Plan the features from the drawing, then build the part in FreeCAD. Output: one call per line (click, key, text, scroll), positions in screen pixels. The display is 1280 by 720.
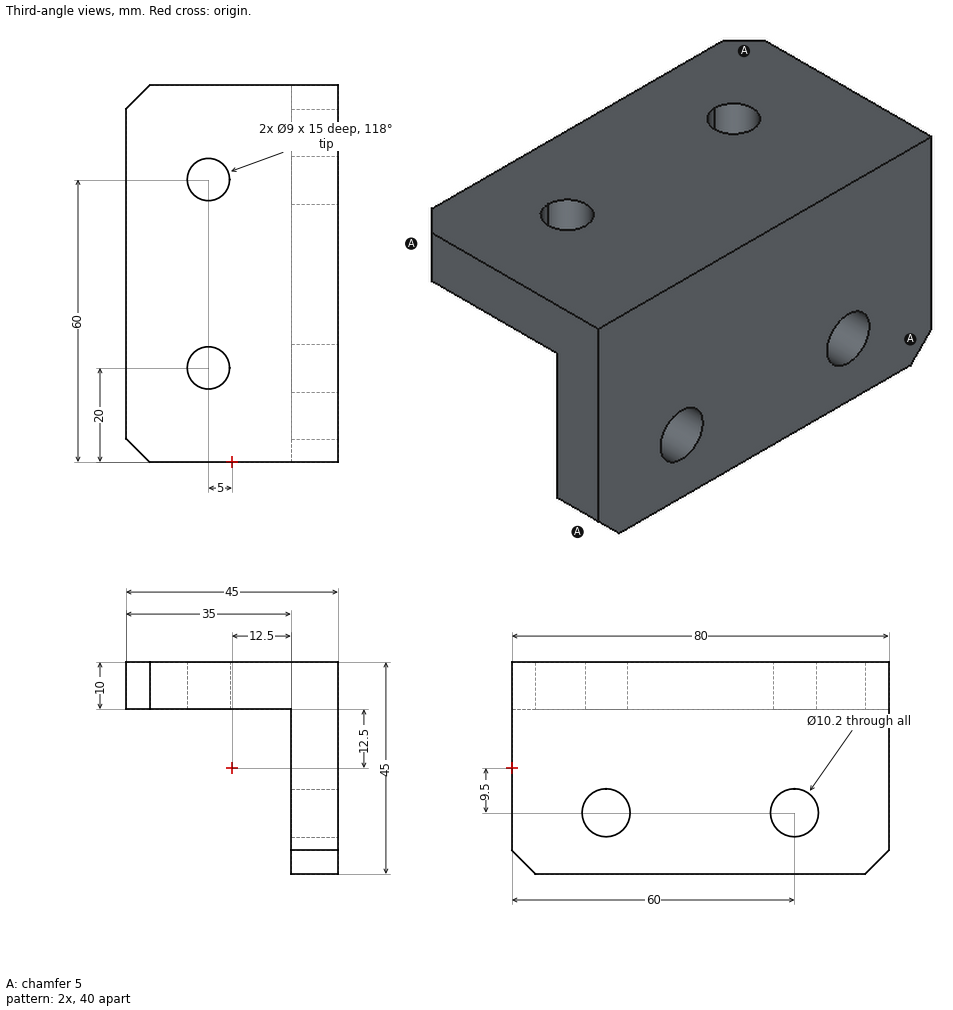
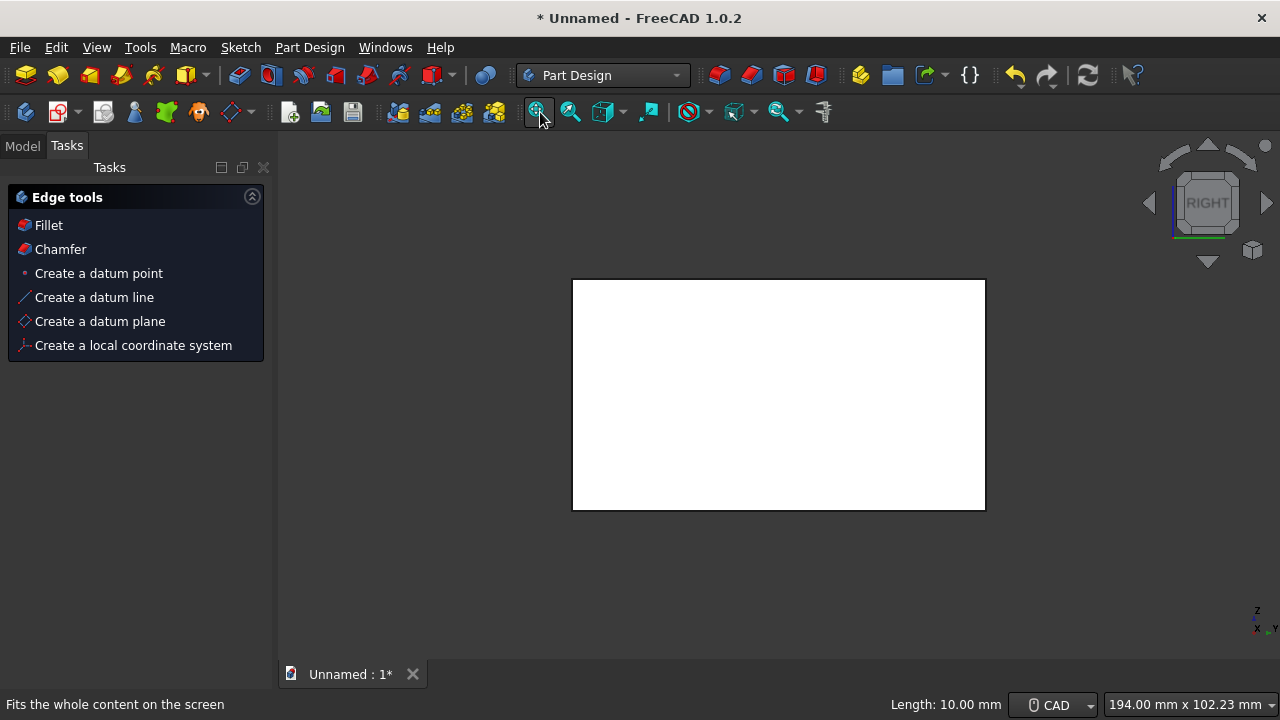
key(5)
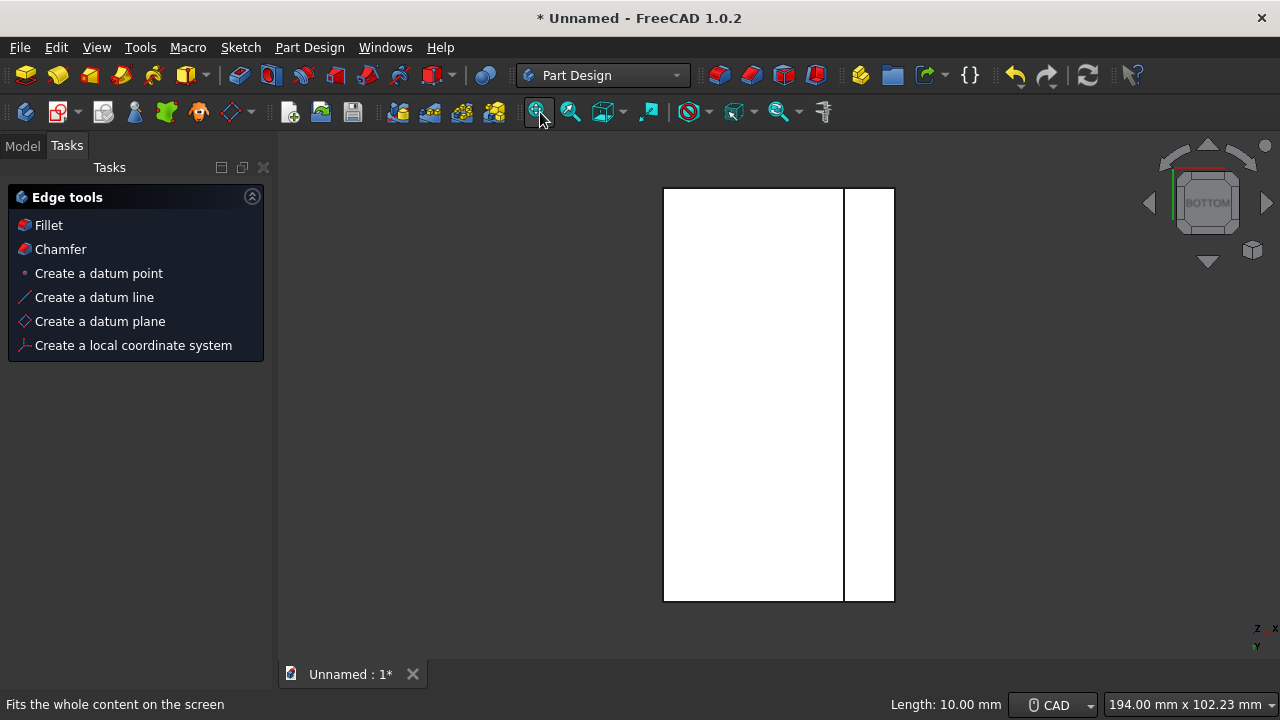
click(869, 187, ctrl)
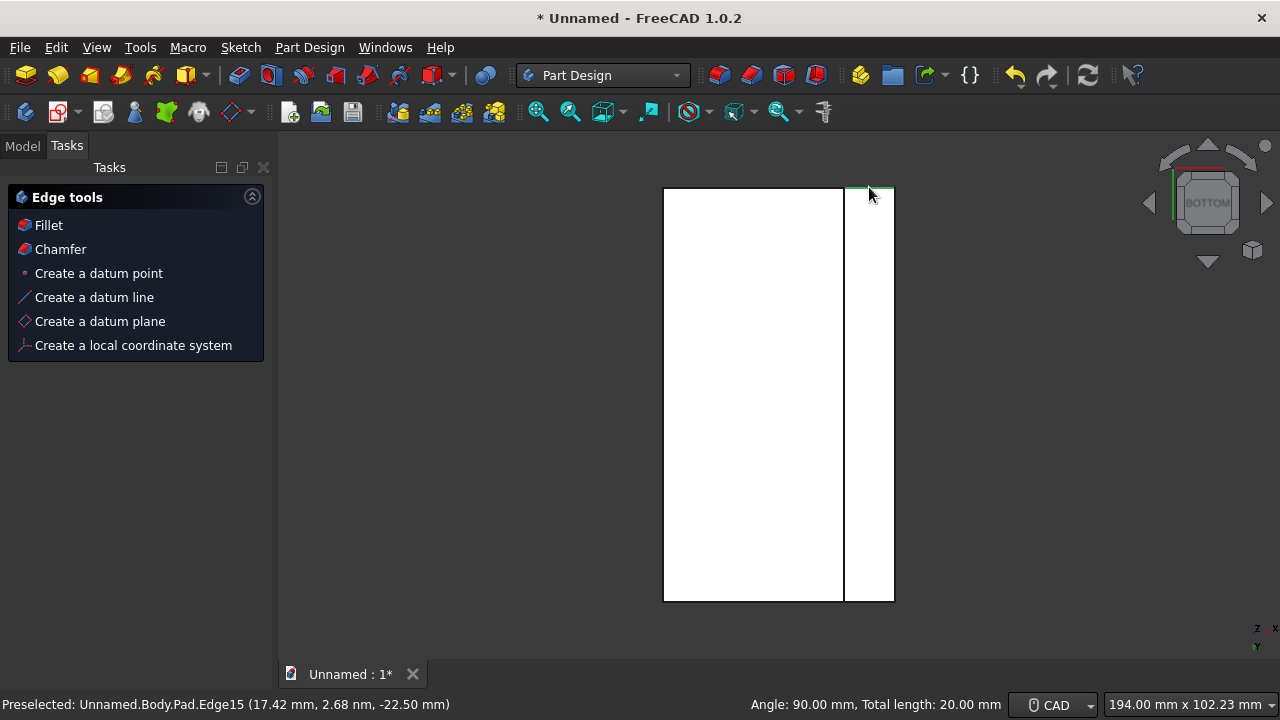
key(4)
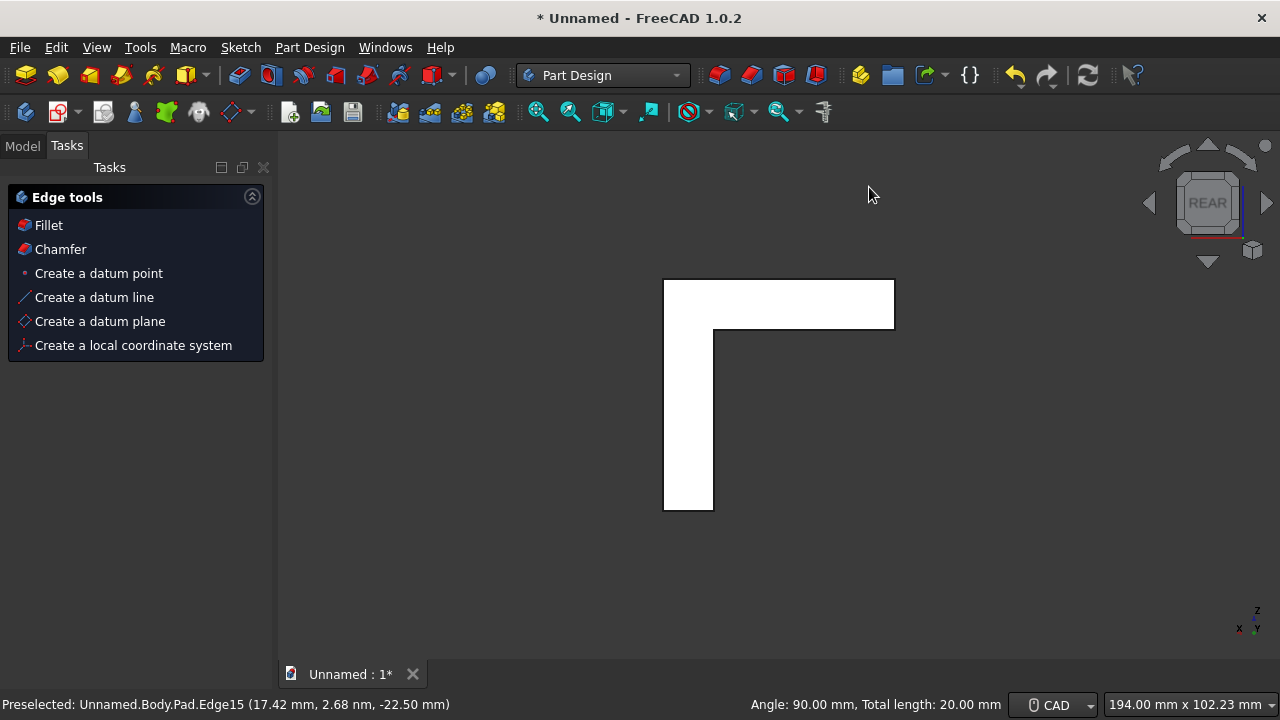
click(540, 112)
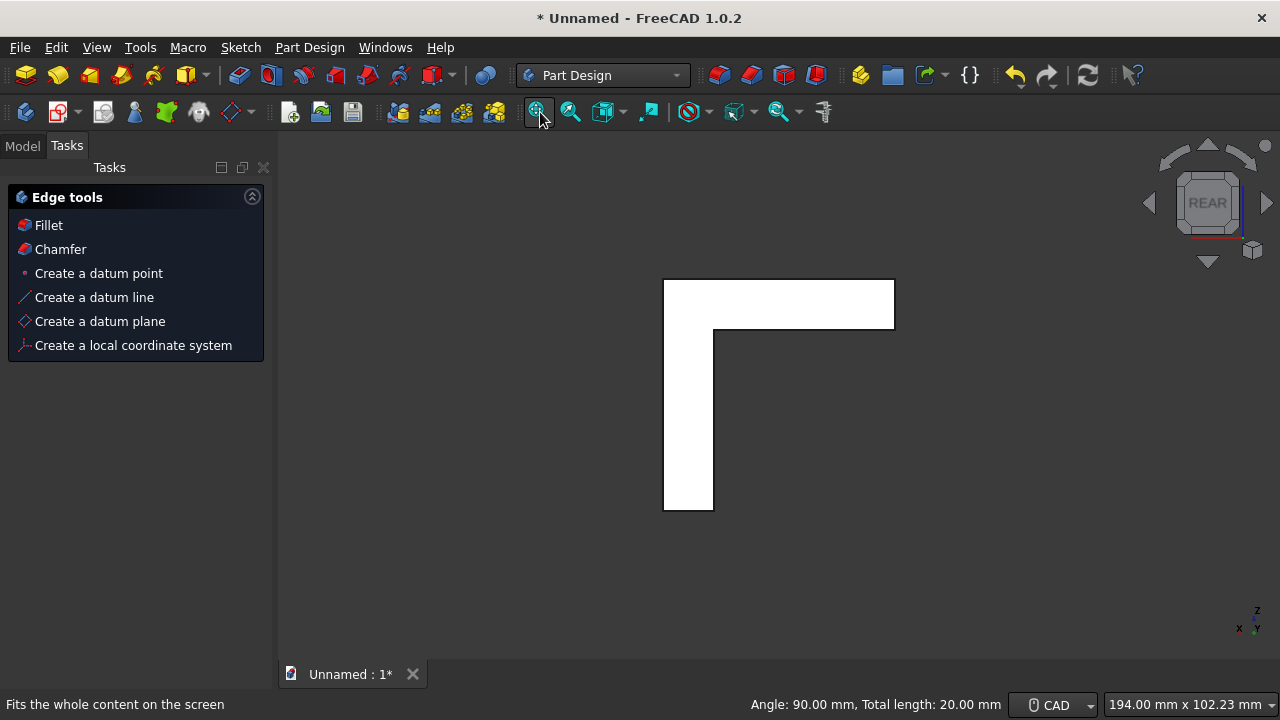
click(895, 304, ctrl)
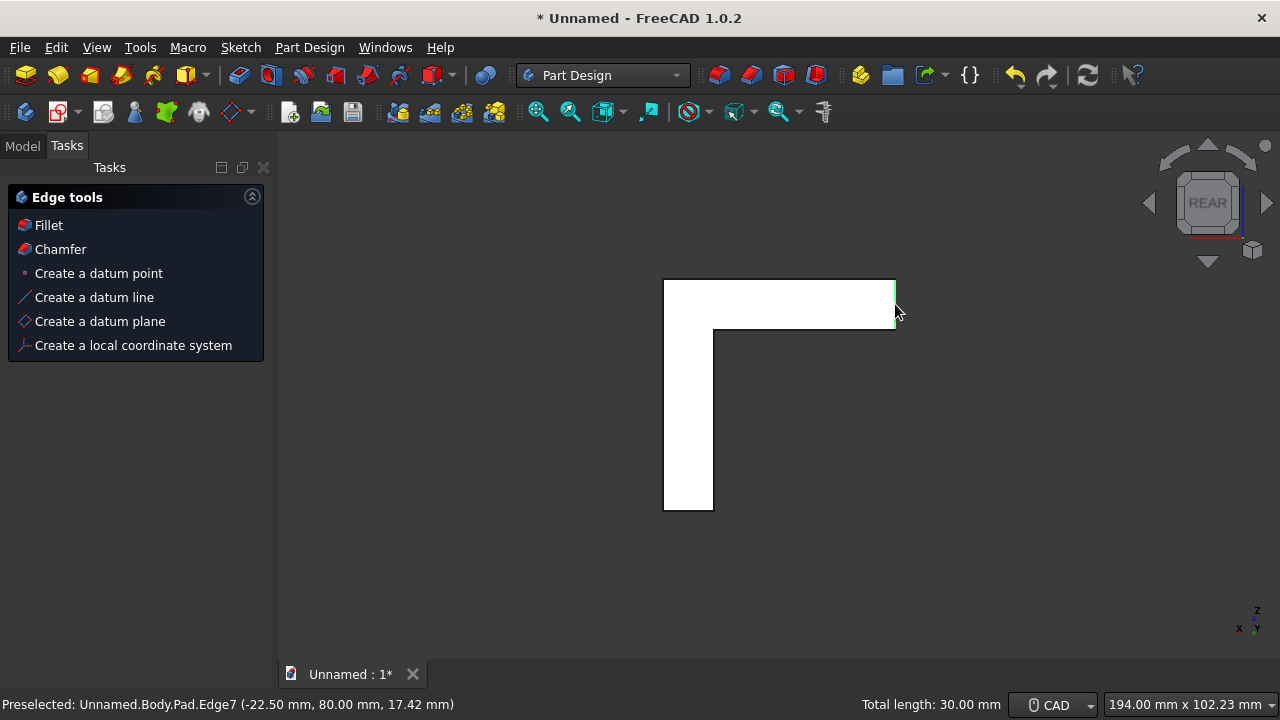
click(689, 510, ctrl)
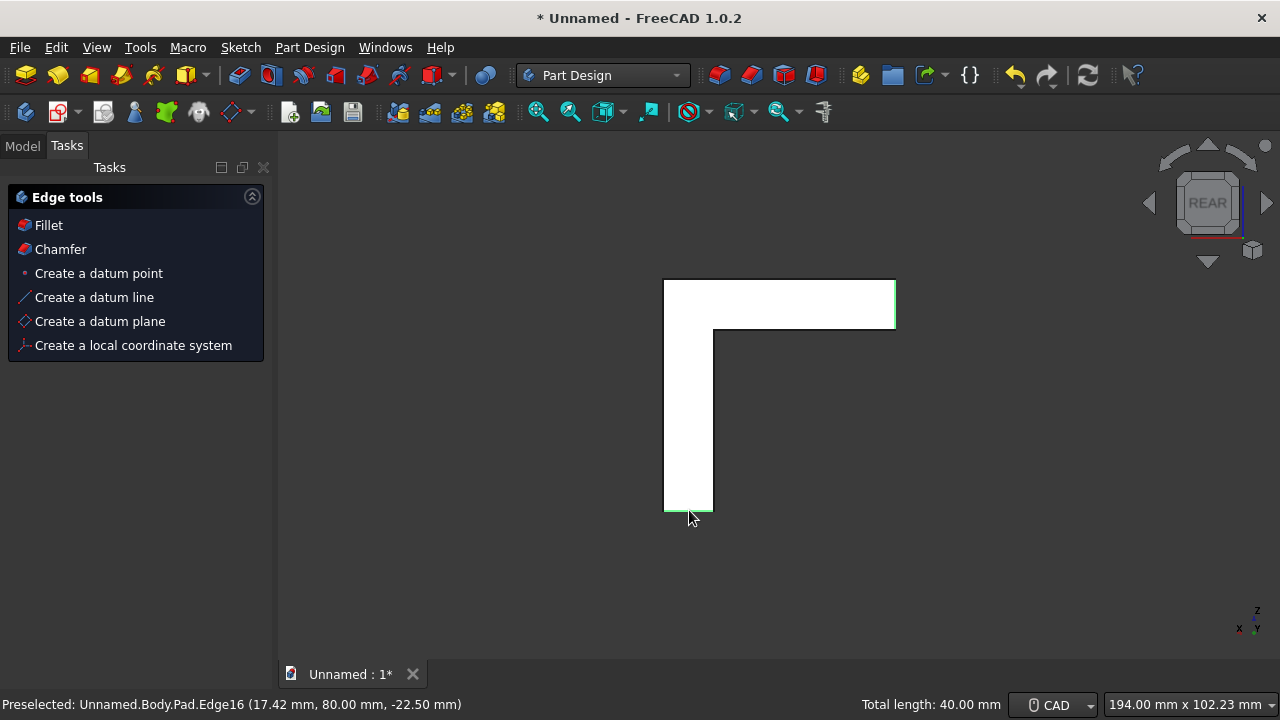
click(752, 76)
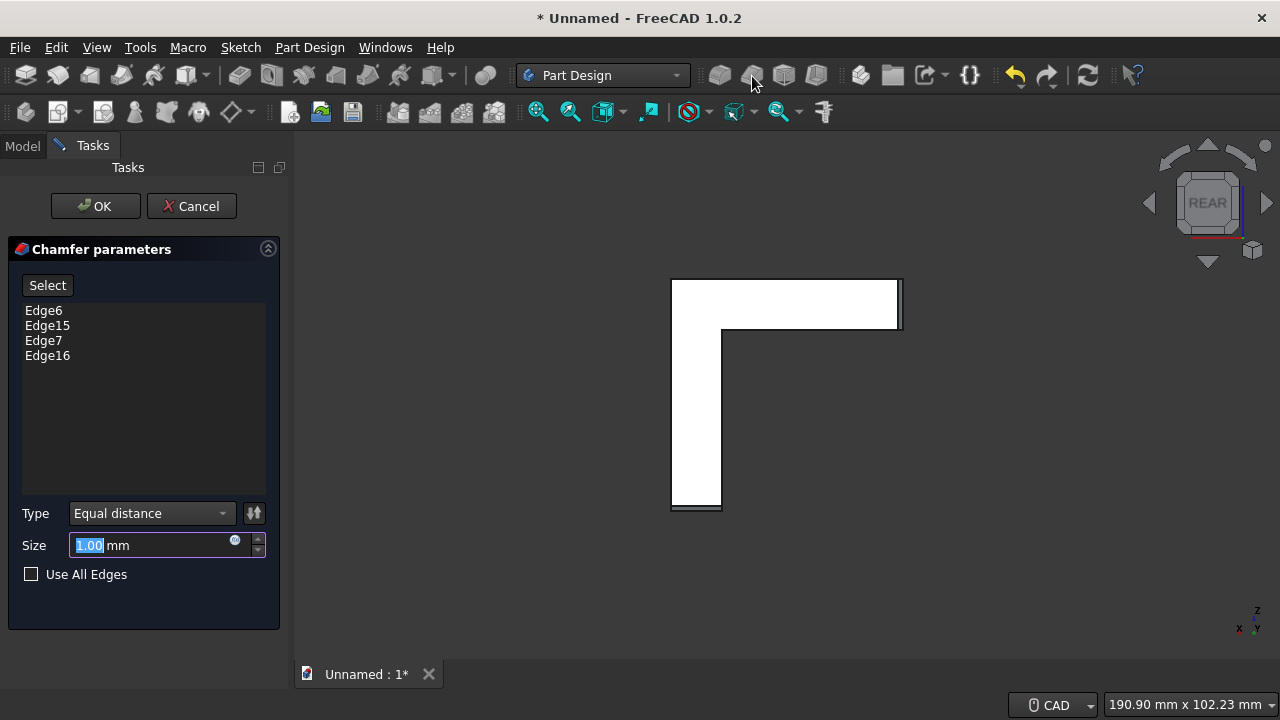
text(5)
key(Tab)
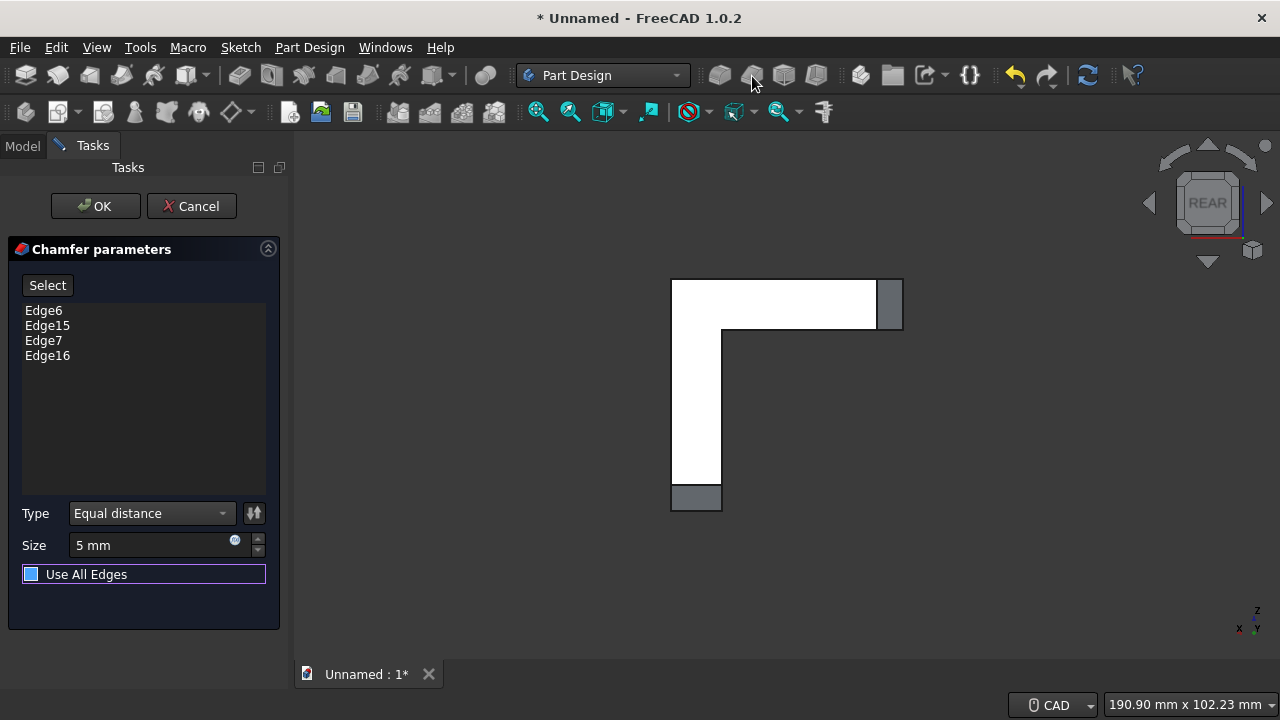
click(96, 206)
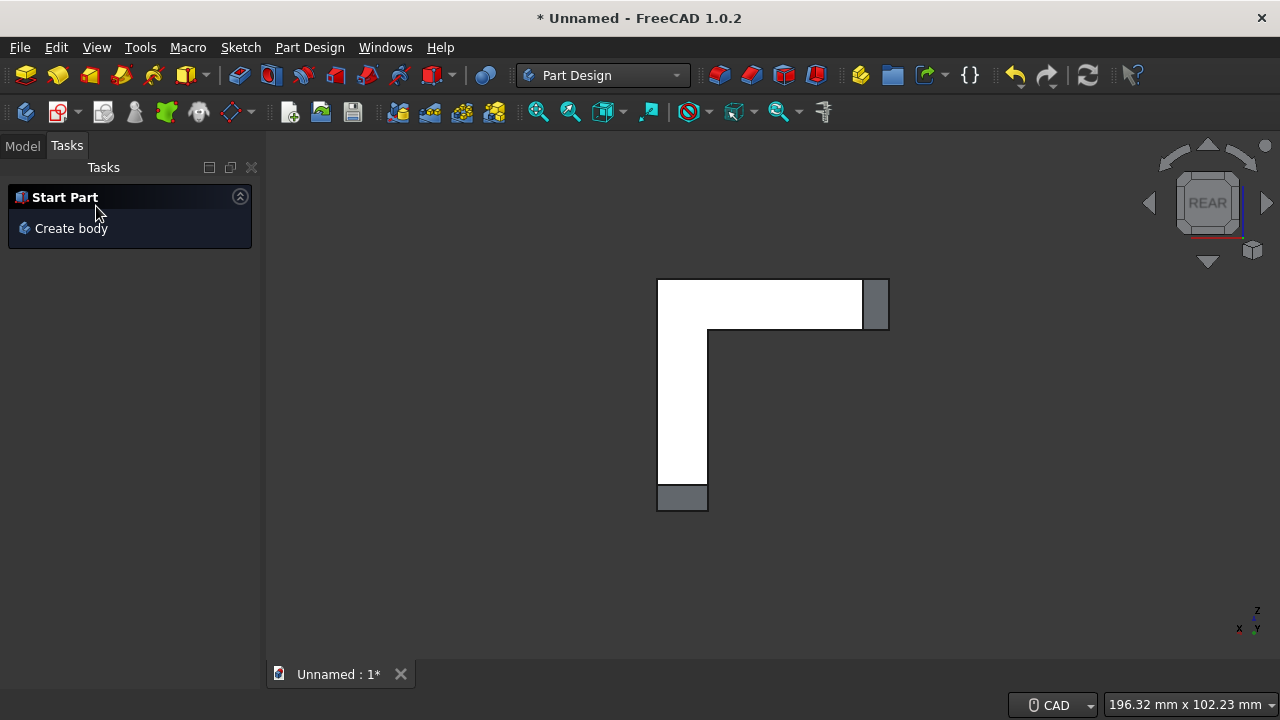
key(v)
key(f)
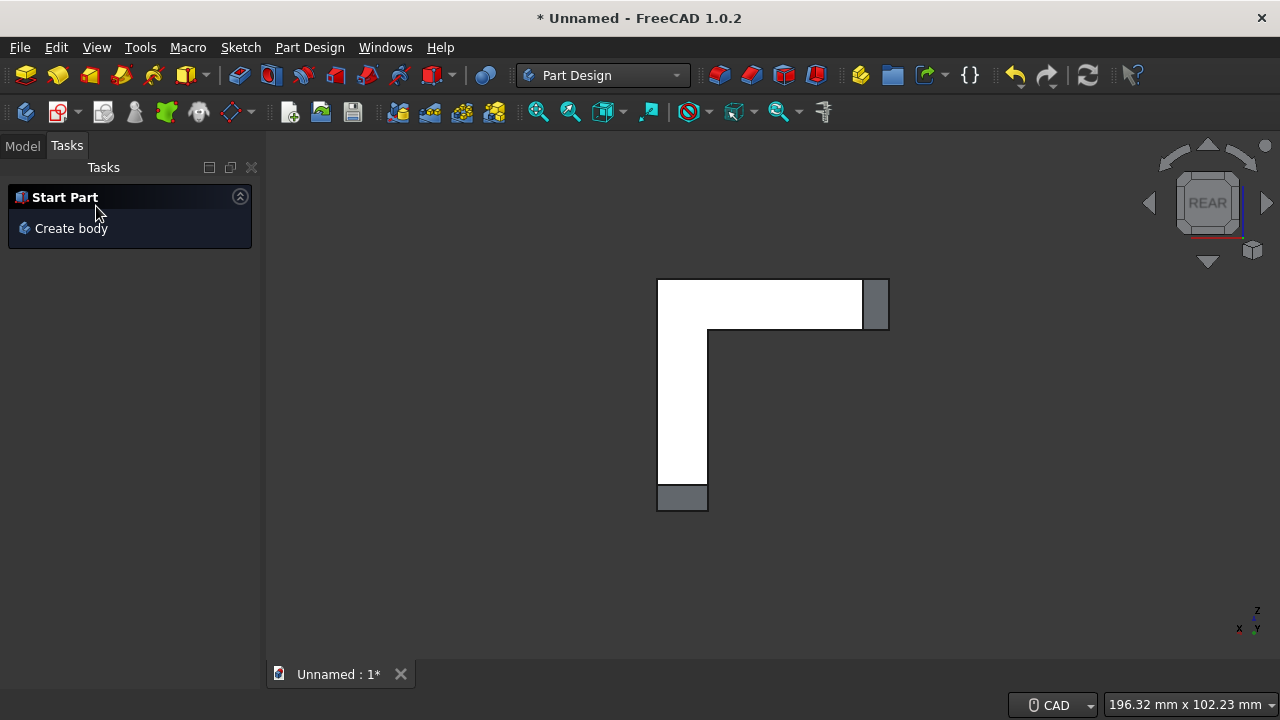
key(5)